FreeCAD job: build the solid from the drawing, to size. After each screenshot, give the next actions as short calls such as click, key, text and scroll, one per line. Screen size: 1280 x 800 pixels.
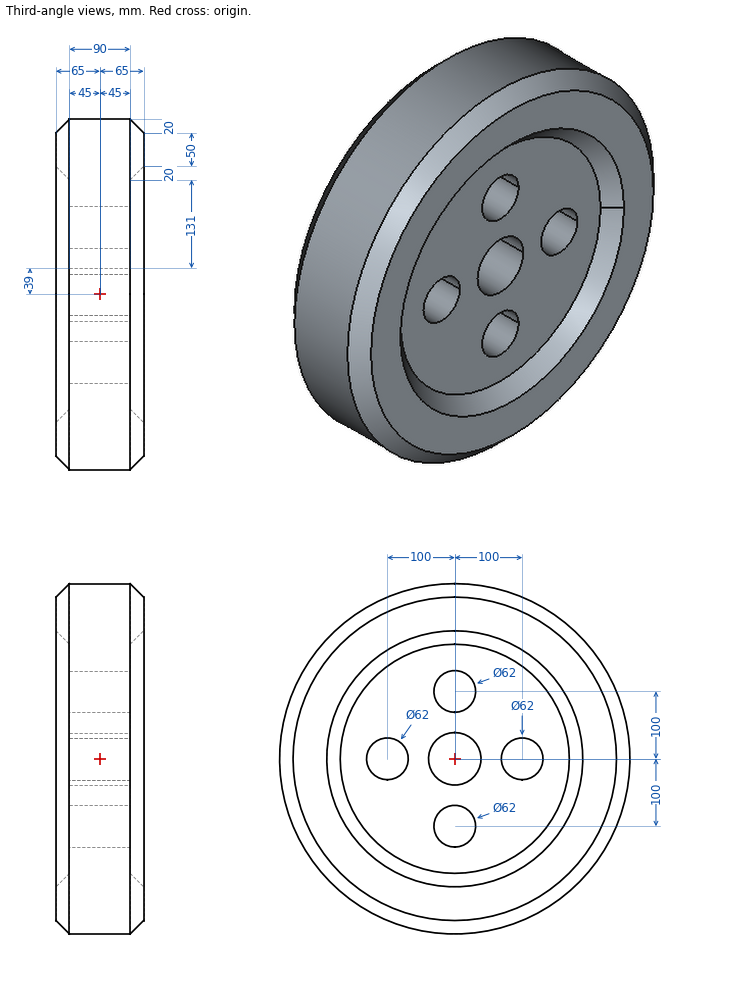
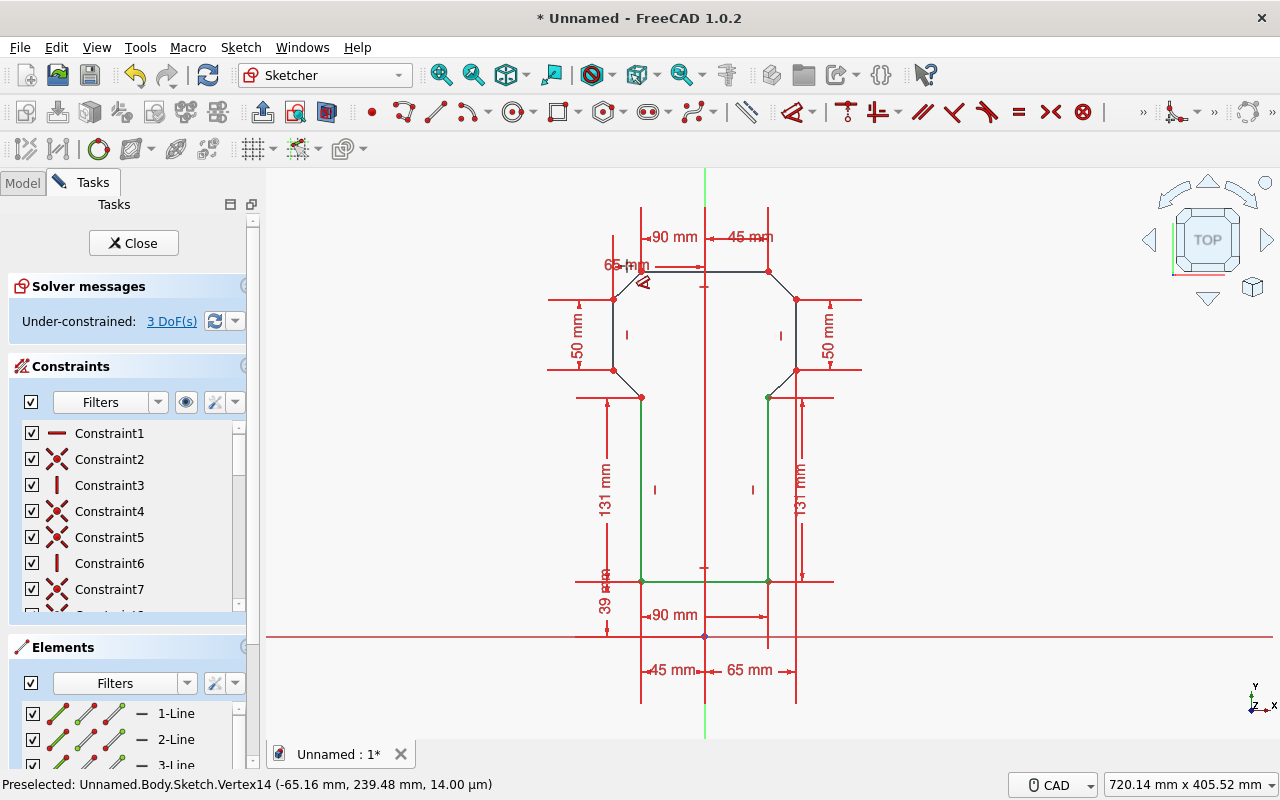
scroll(777, 389, up, 2)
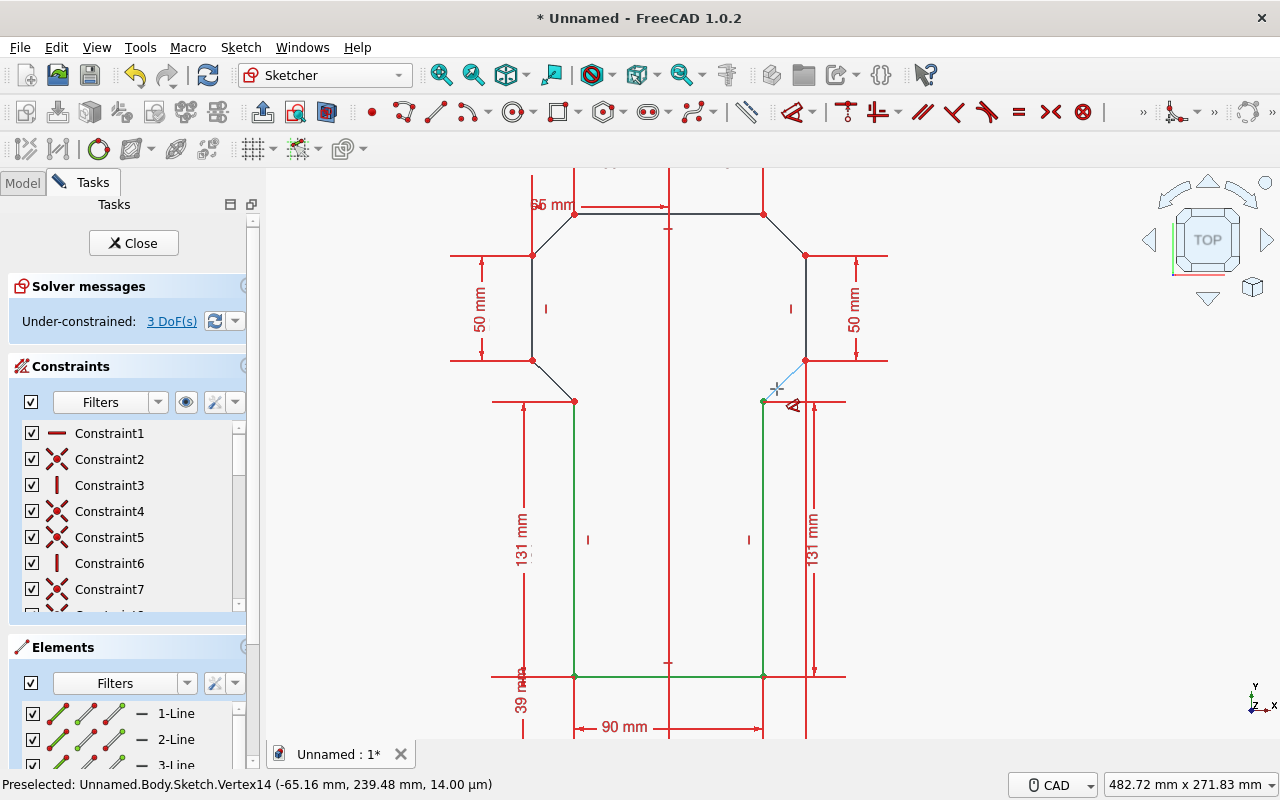
click(776, 389)
click(840, 381)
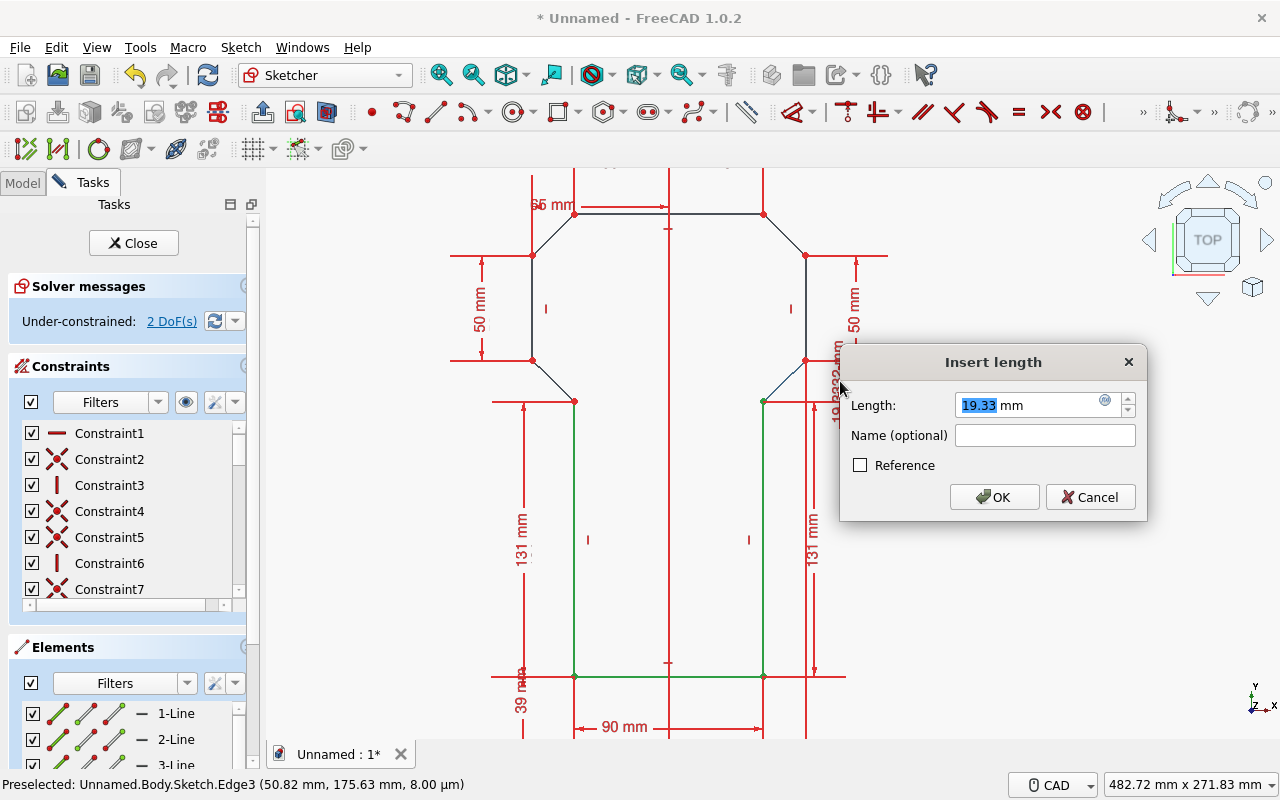
text(20)
key(Return)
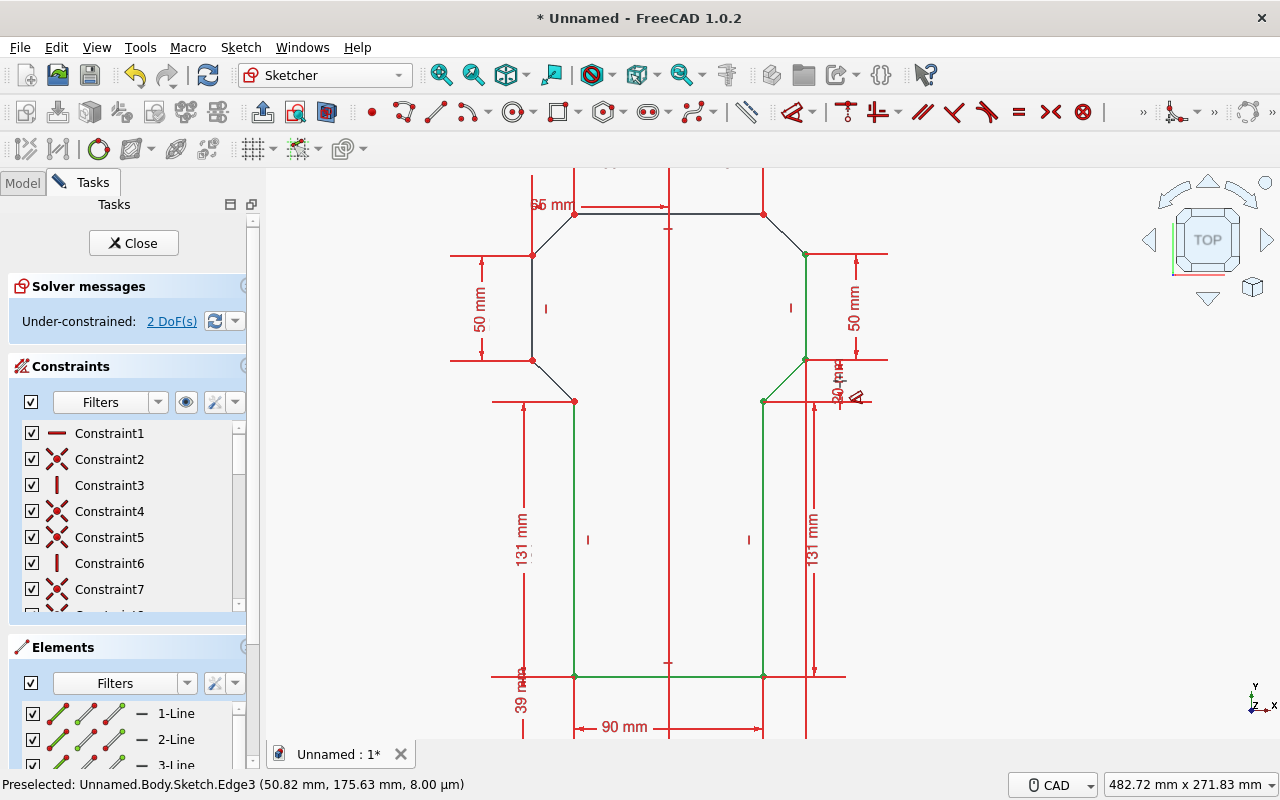
click(793, 242)
click(840, 234)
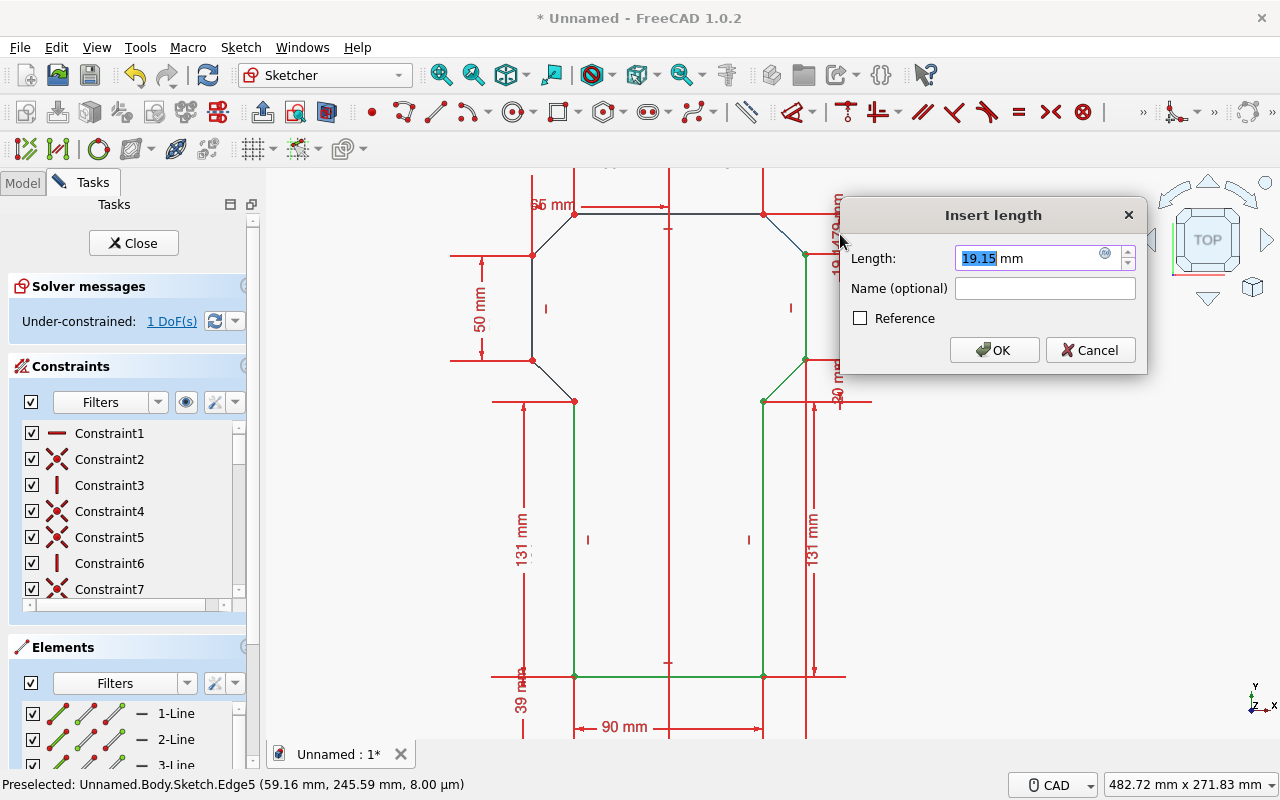
text(20)
key(Return)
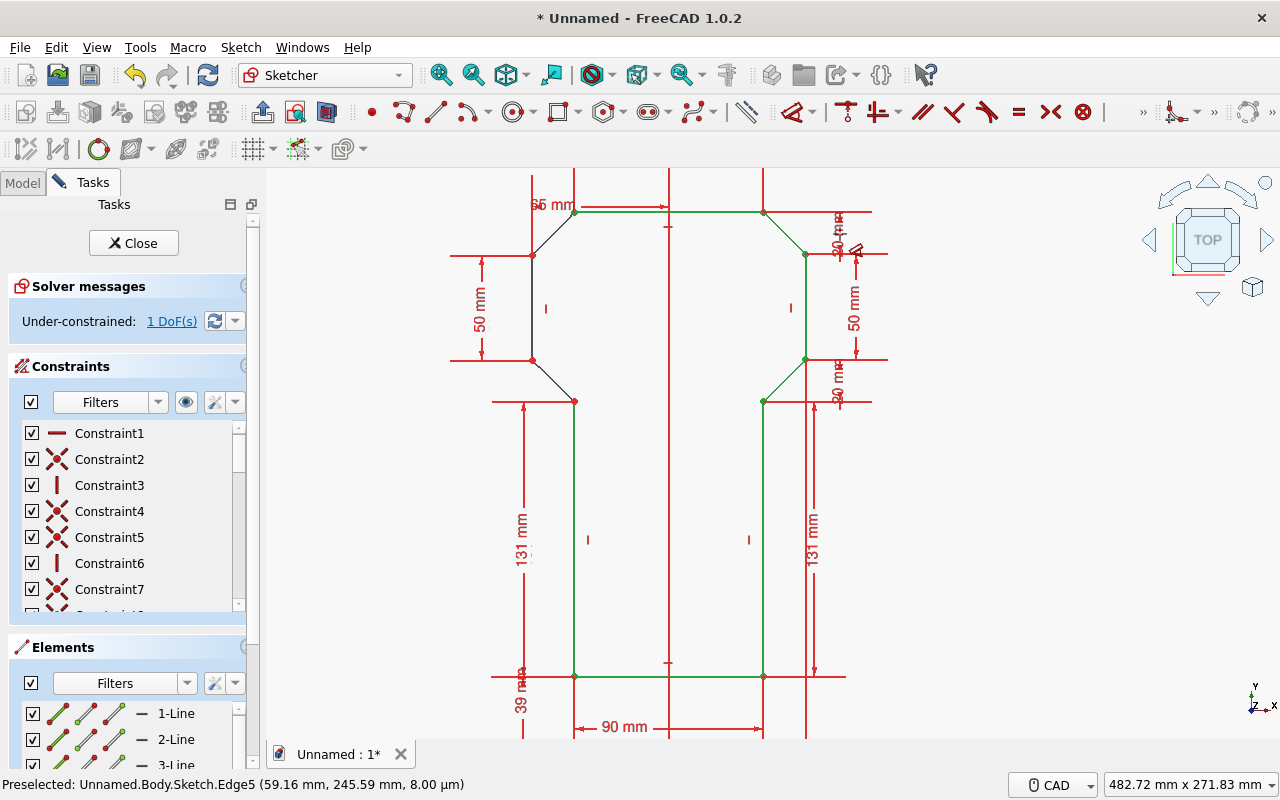
click(562, 225)
click(498, 234)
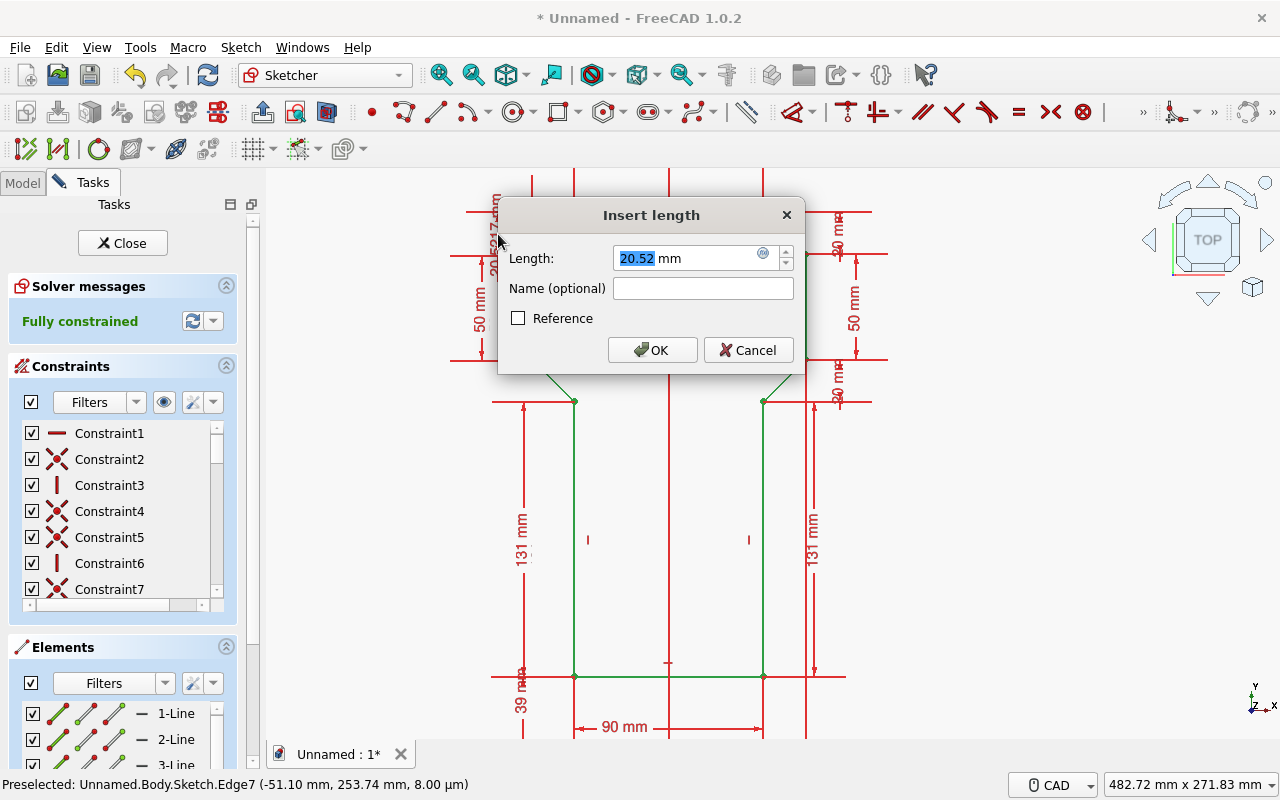
text(20)
key(Return)
key(Escape)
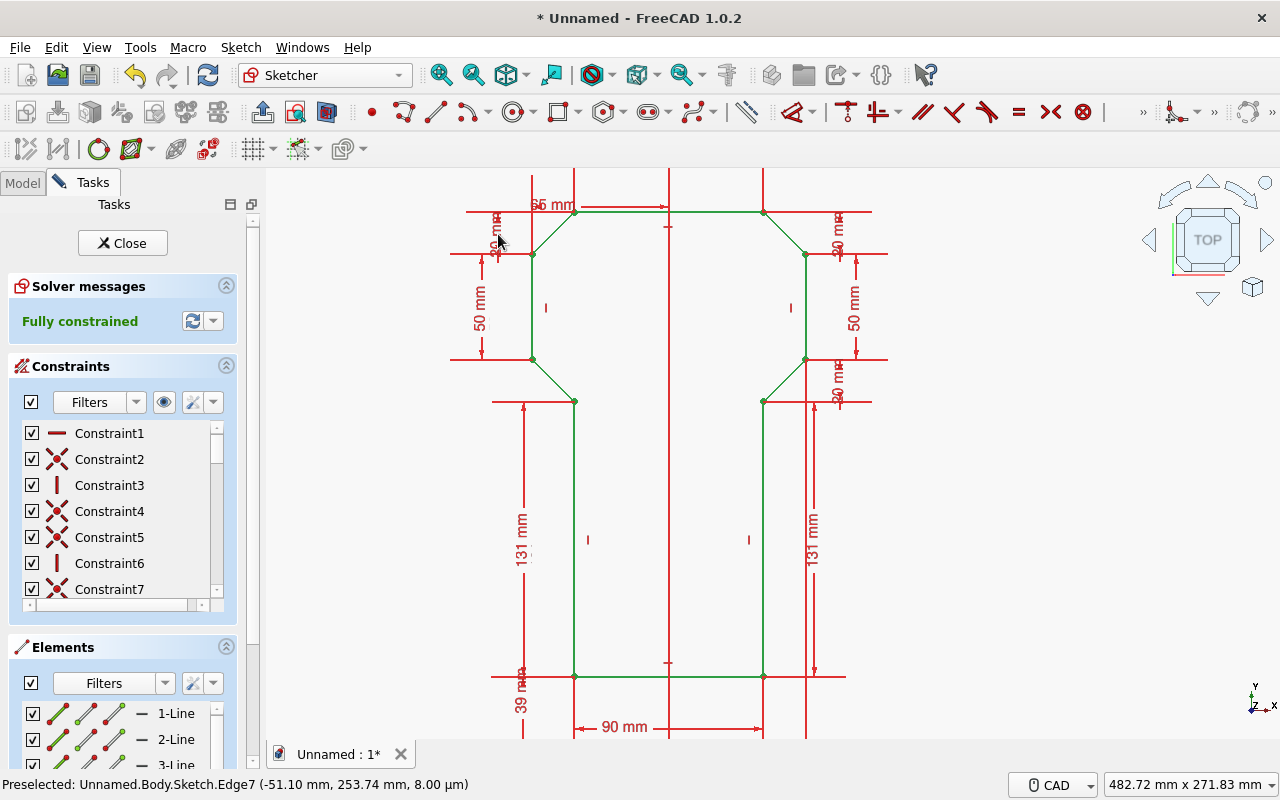
click(123, 243)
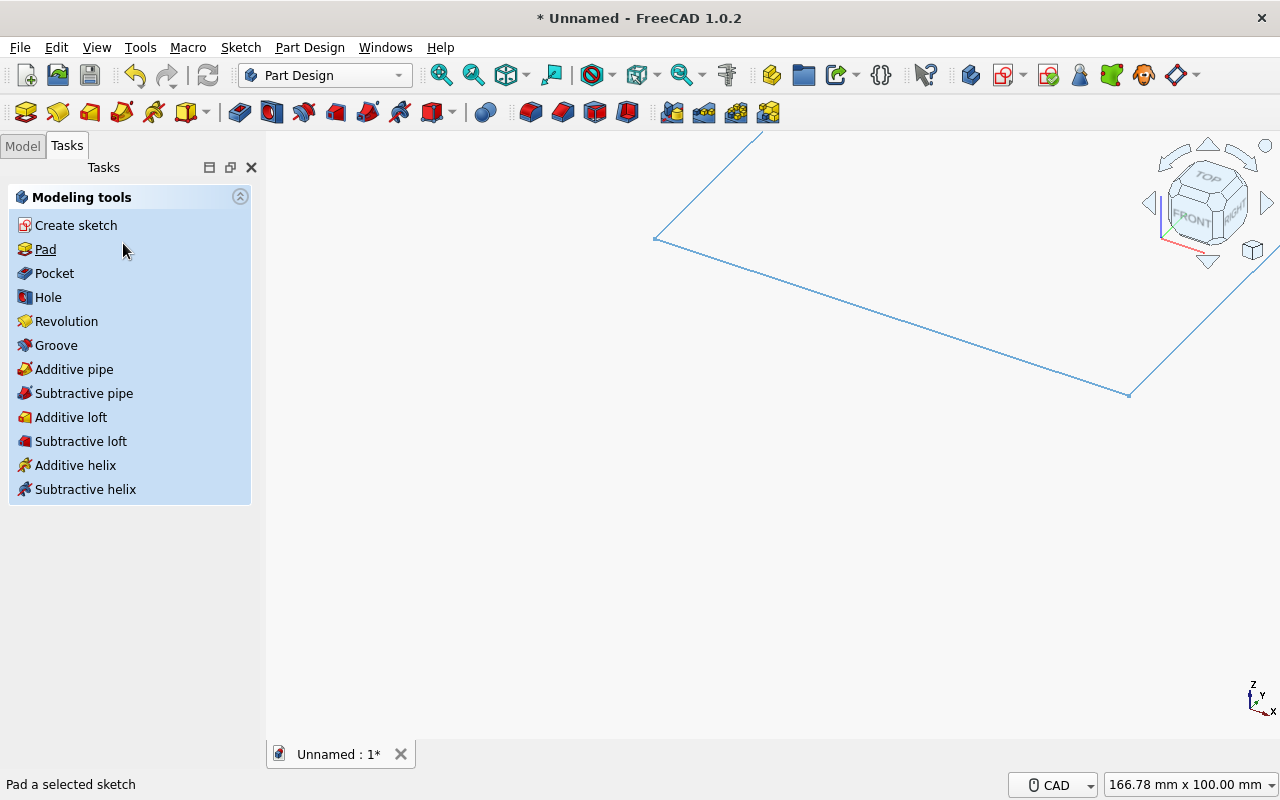
click(58, 112)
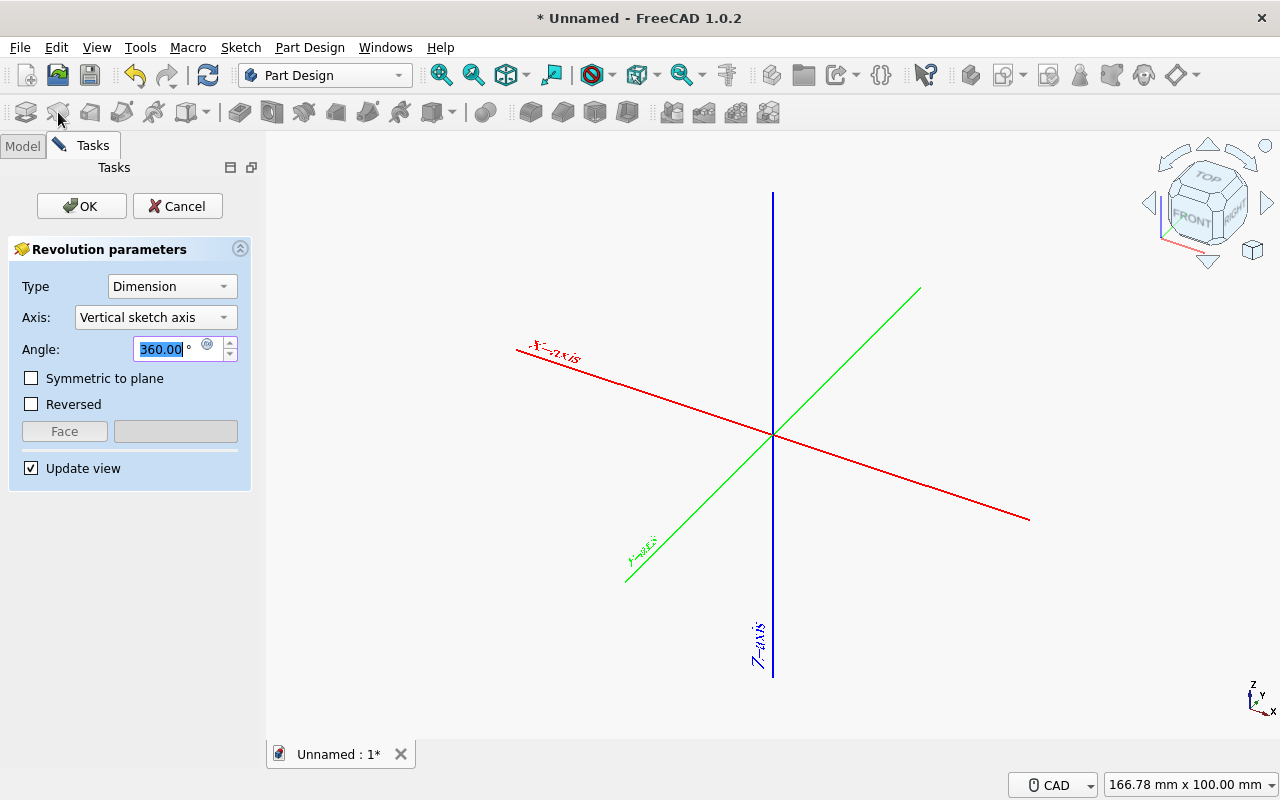
click(156, 318)